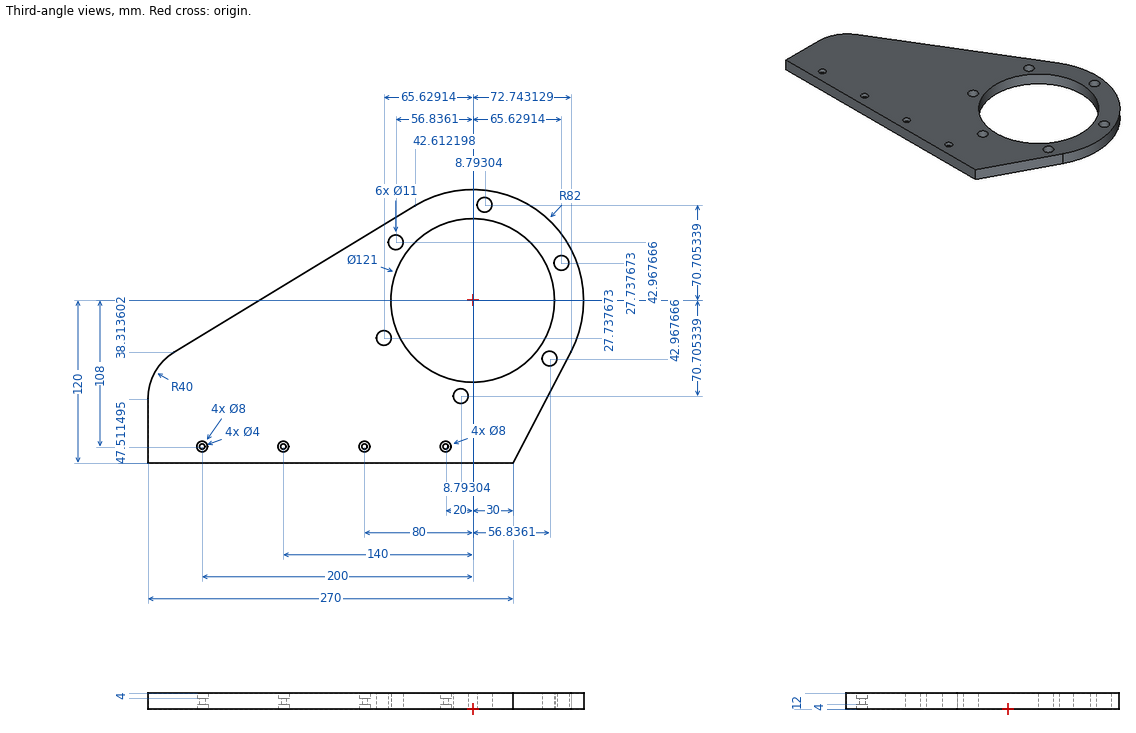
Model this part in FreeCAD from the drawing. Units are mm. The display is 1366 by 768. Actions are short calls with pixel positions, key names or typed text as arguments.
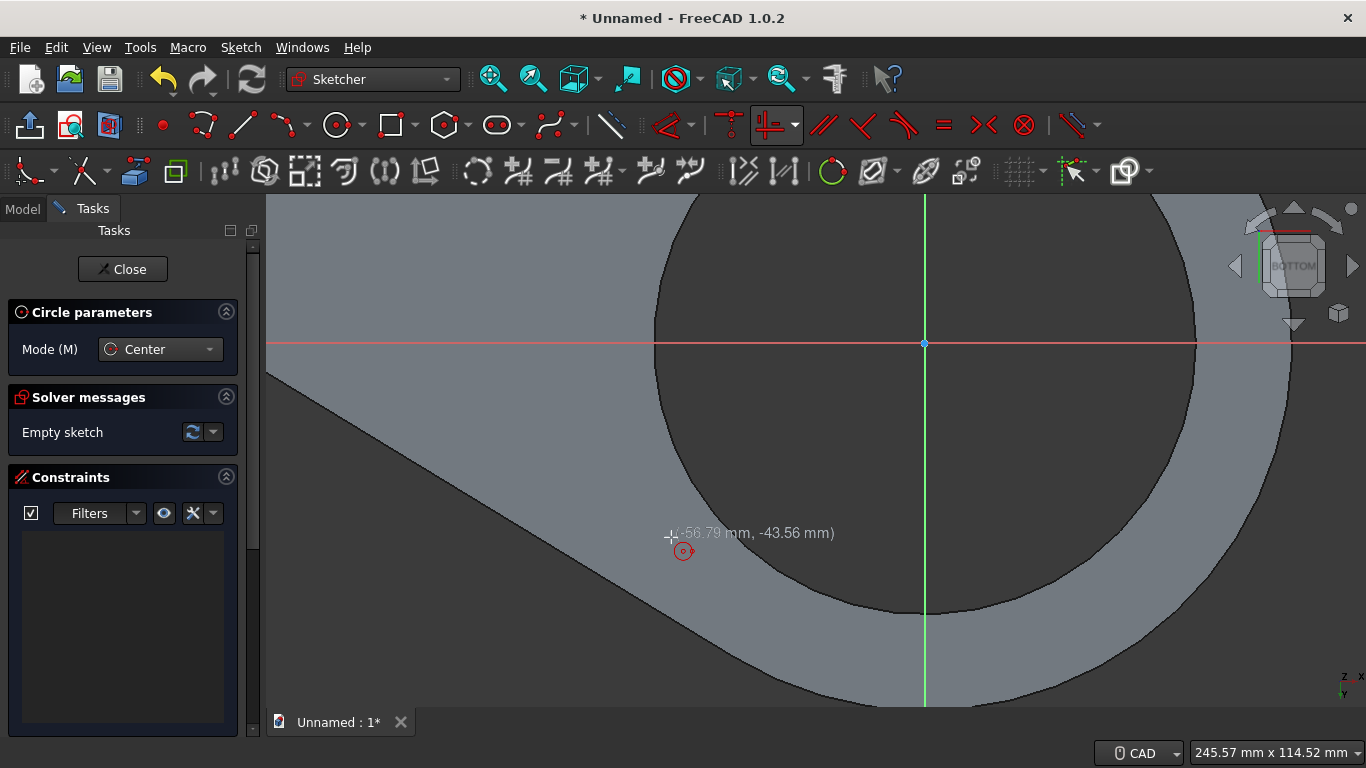
click(670, 536)
click(688, 518)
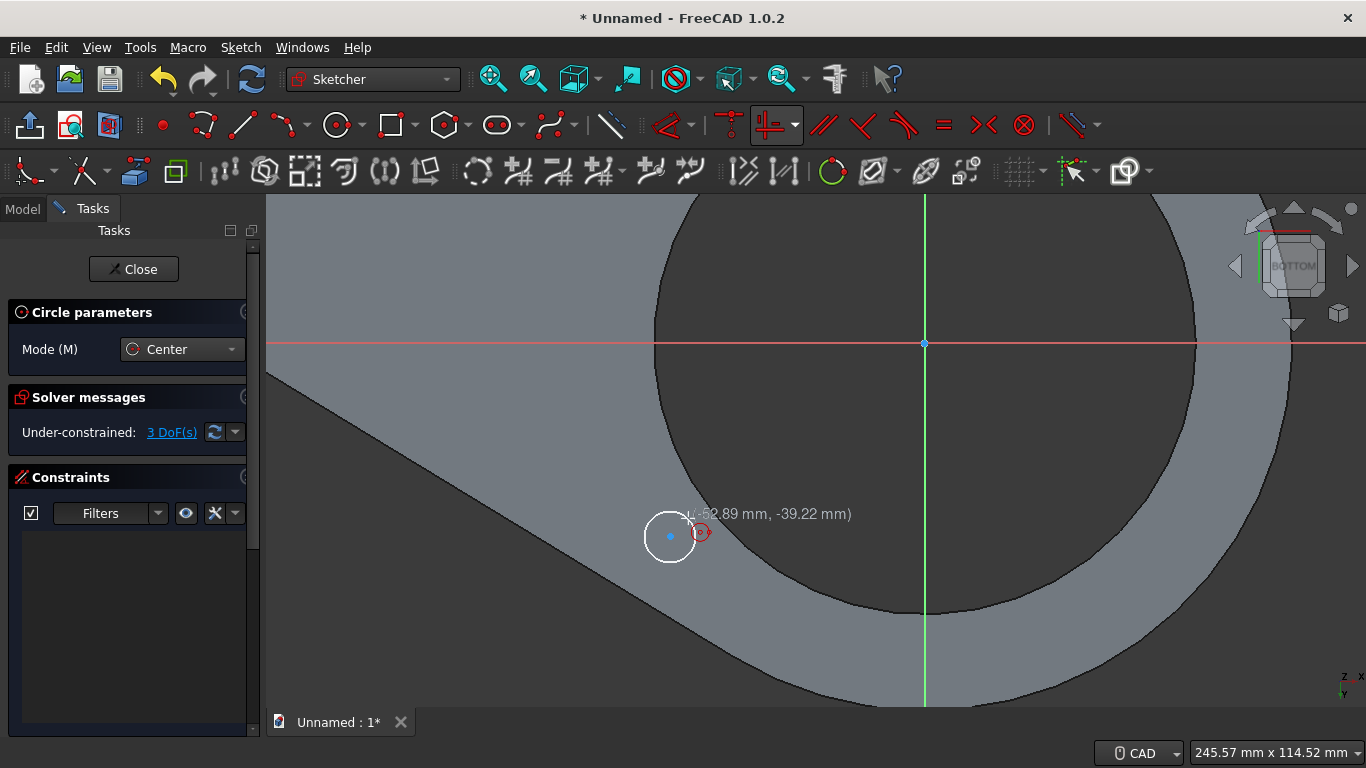
click(964, 660)
click(982, 643)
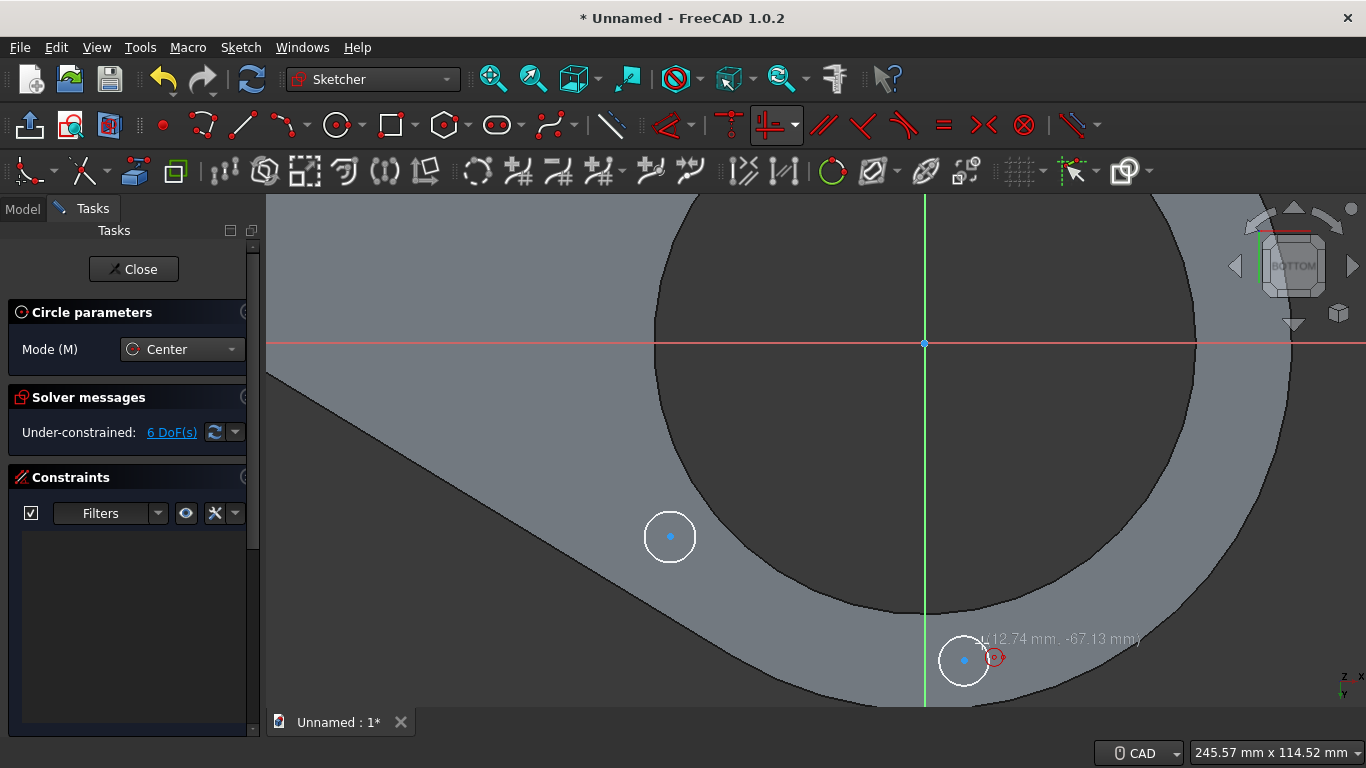
scroll(603, 538, down, 4)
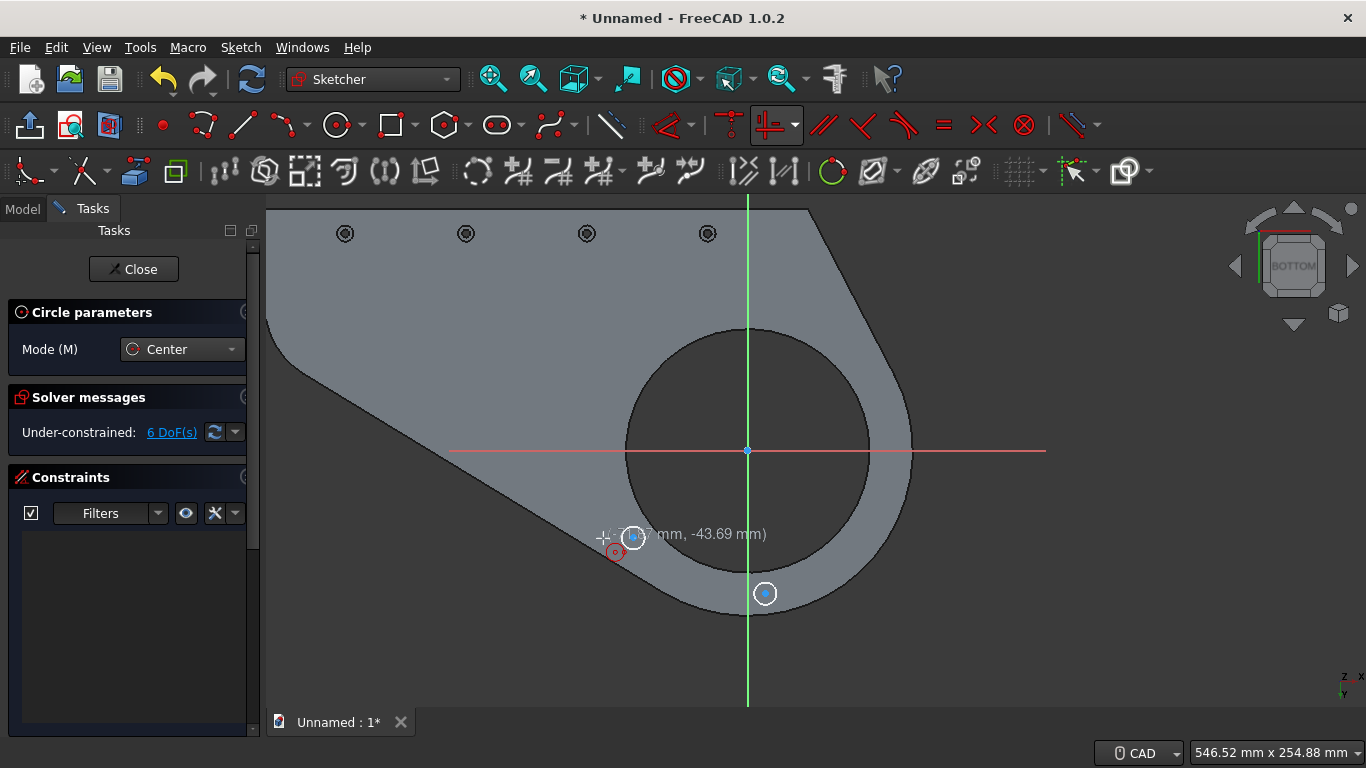
scroll(616, 395, up, 4)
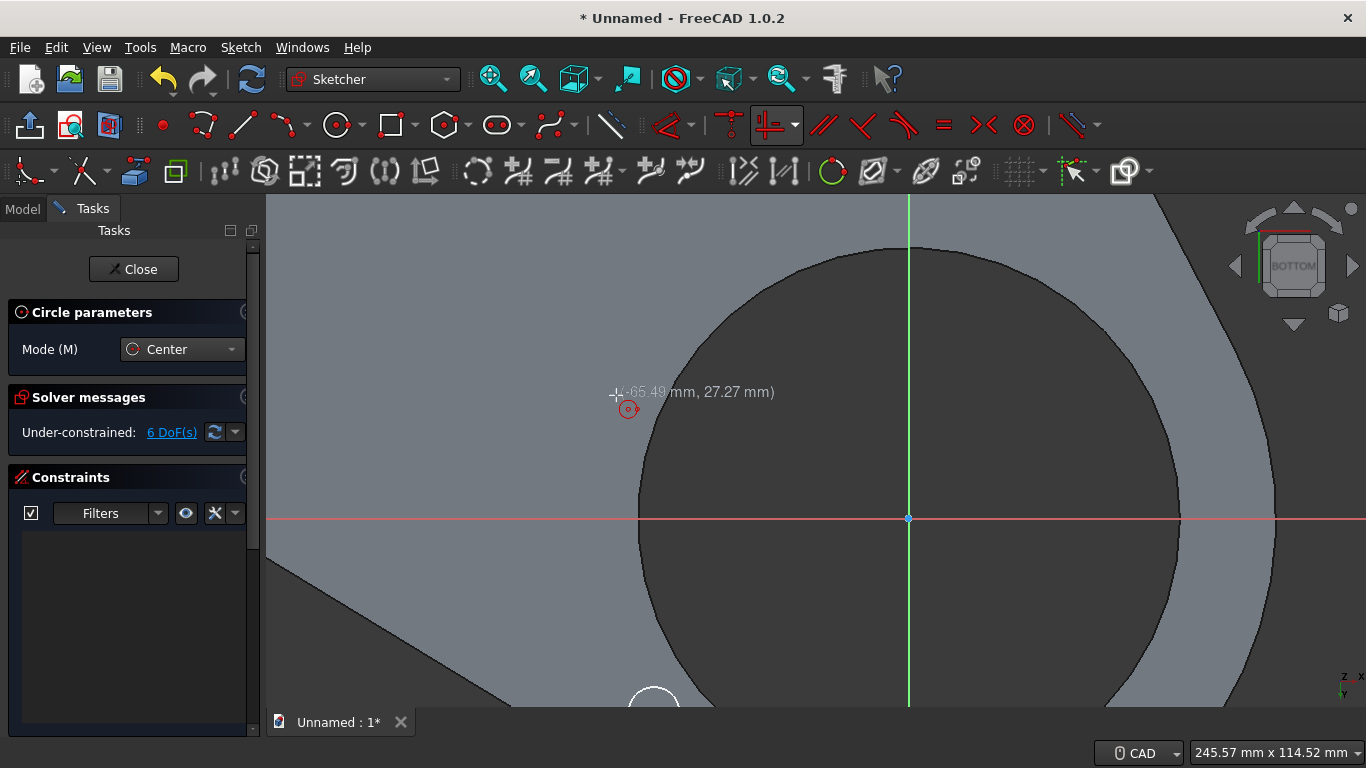
click(615, 395)
click(632, 377)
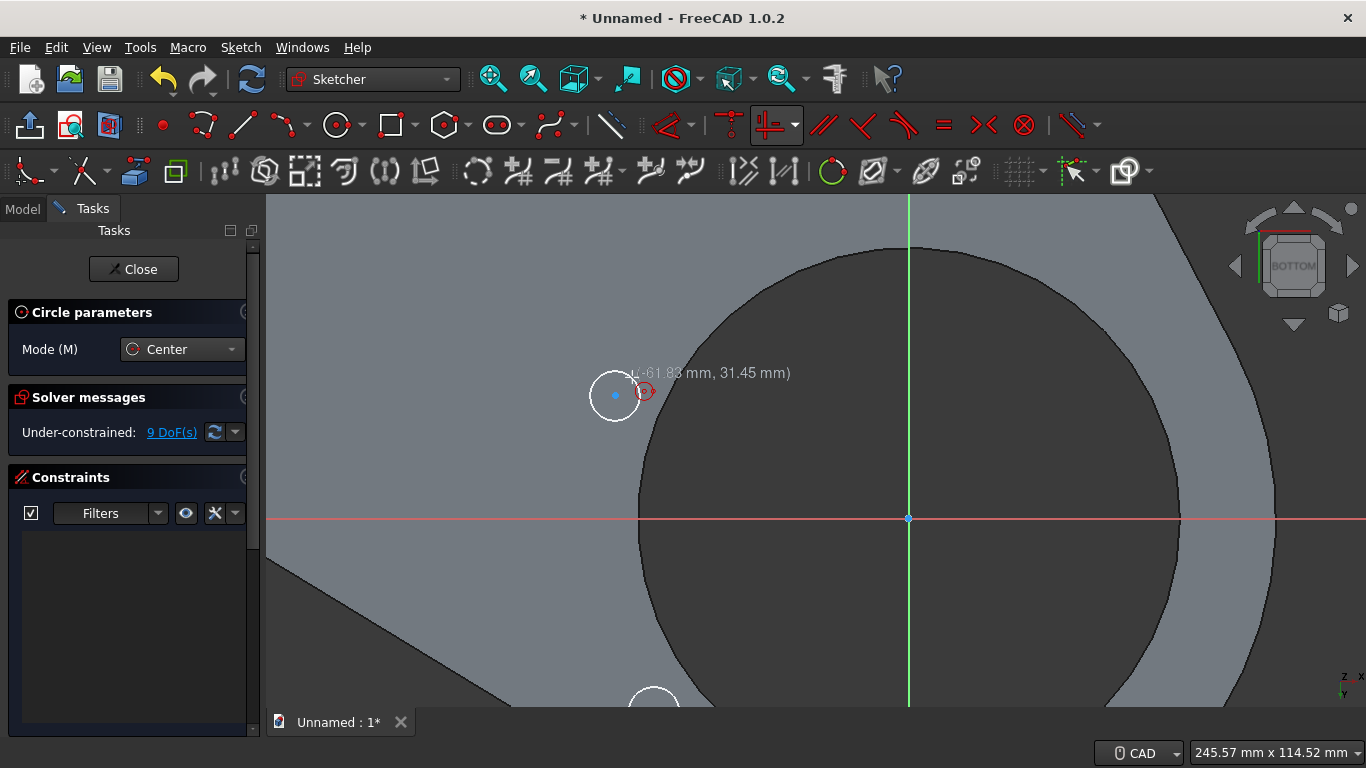
scroll(616, 395, down, 4)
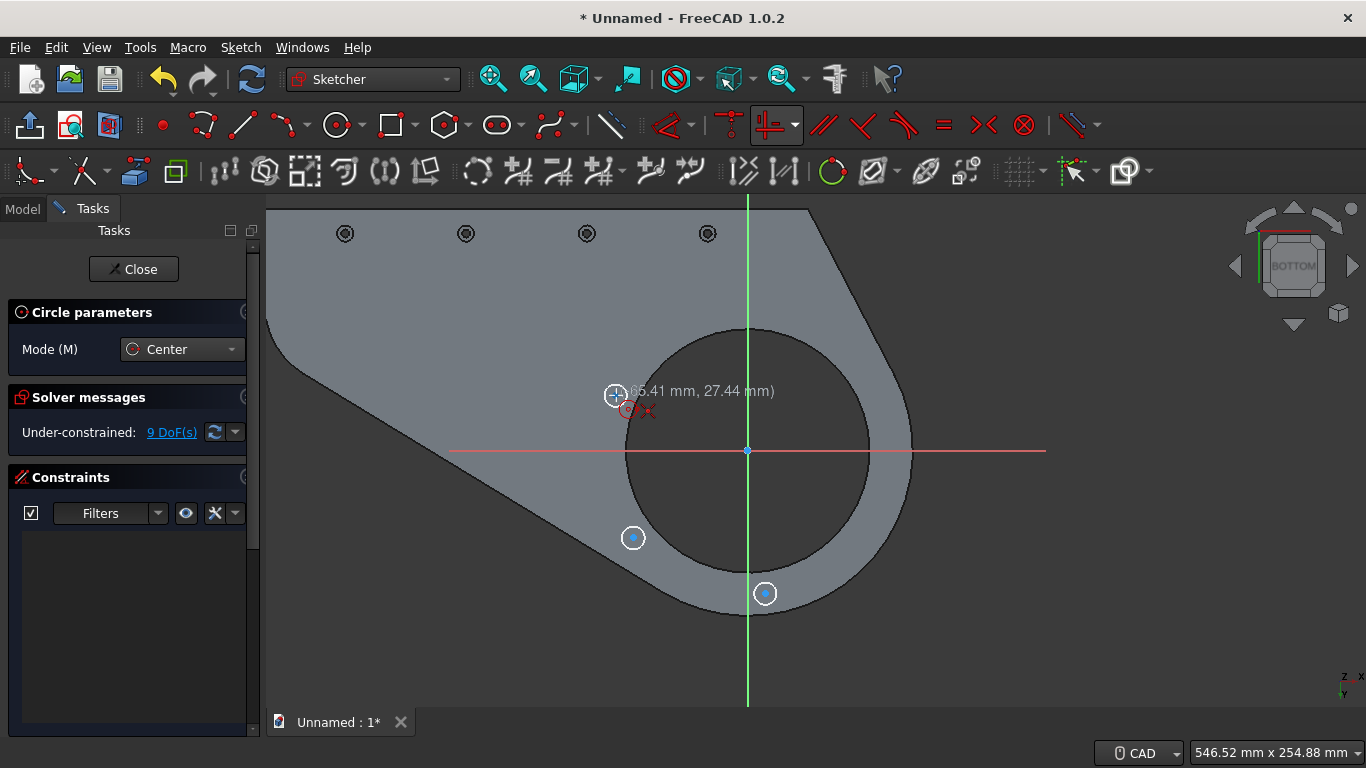
scroll(730, 309, up, 4)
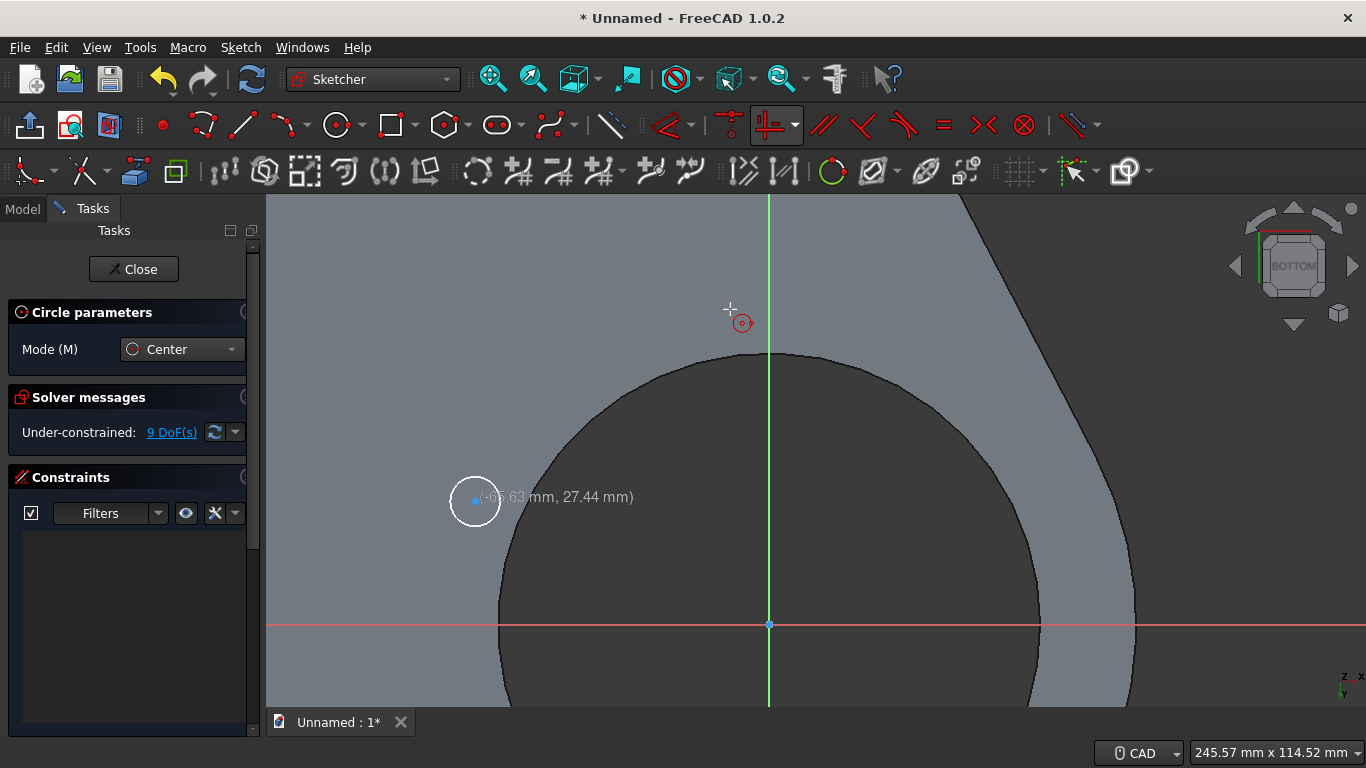
click(730, 308)
click(747, 290)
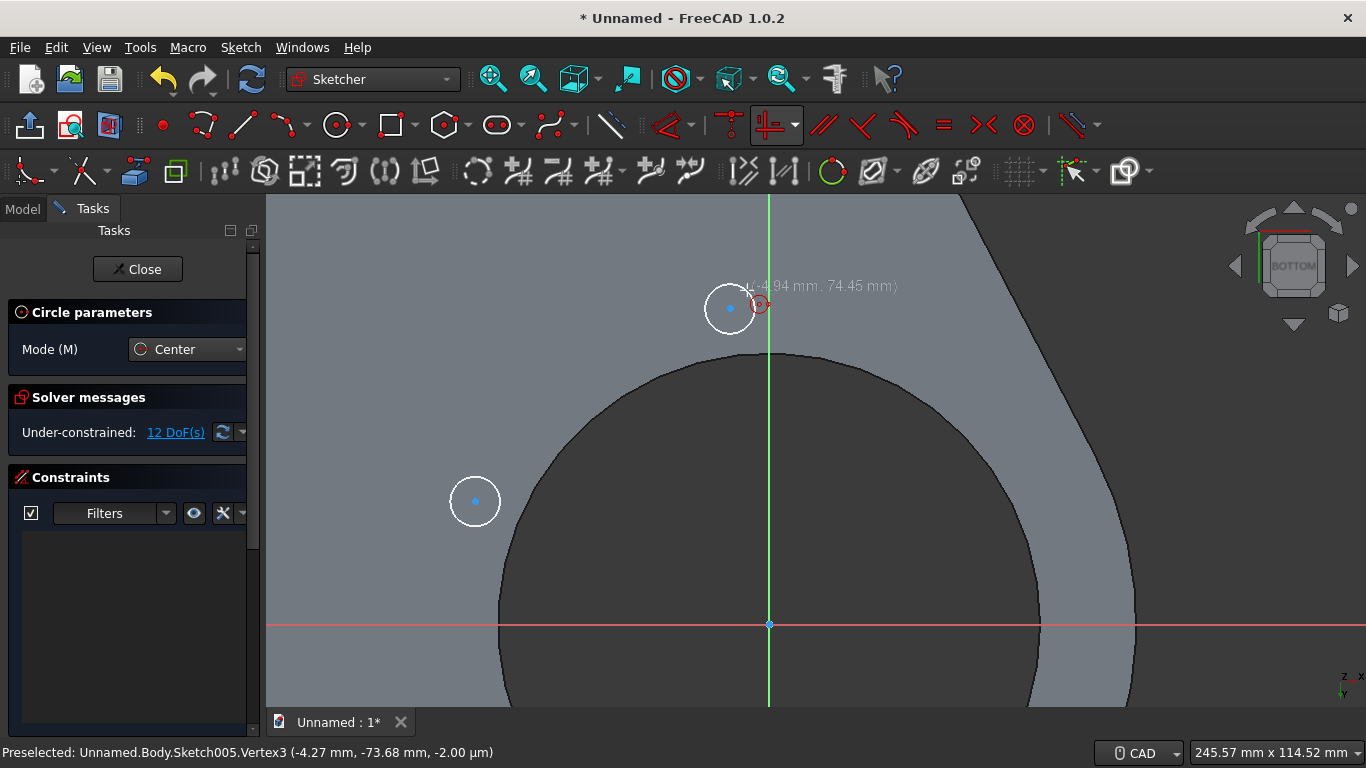
click(1024, 432)
click(1041, 415)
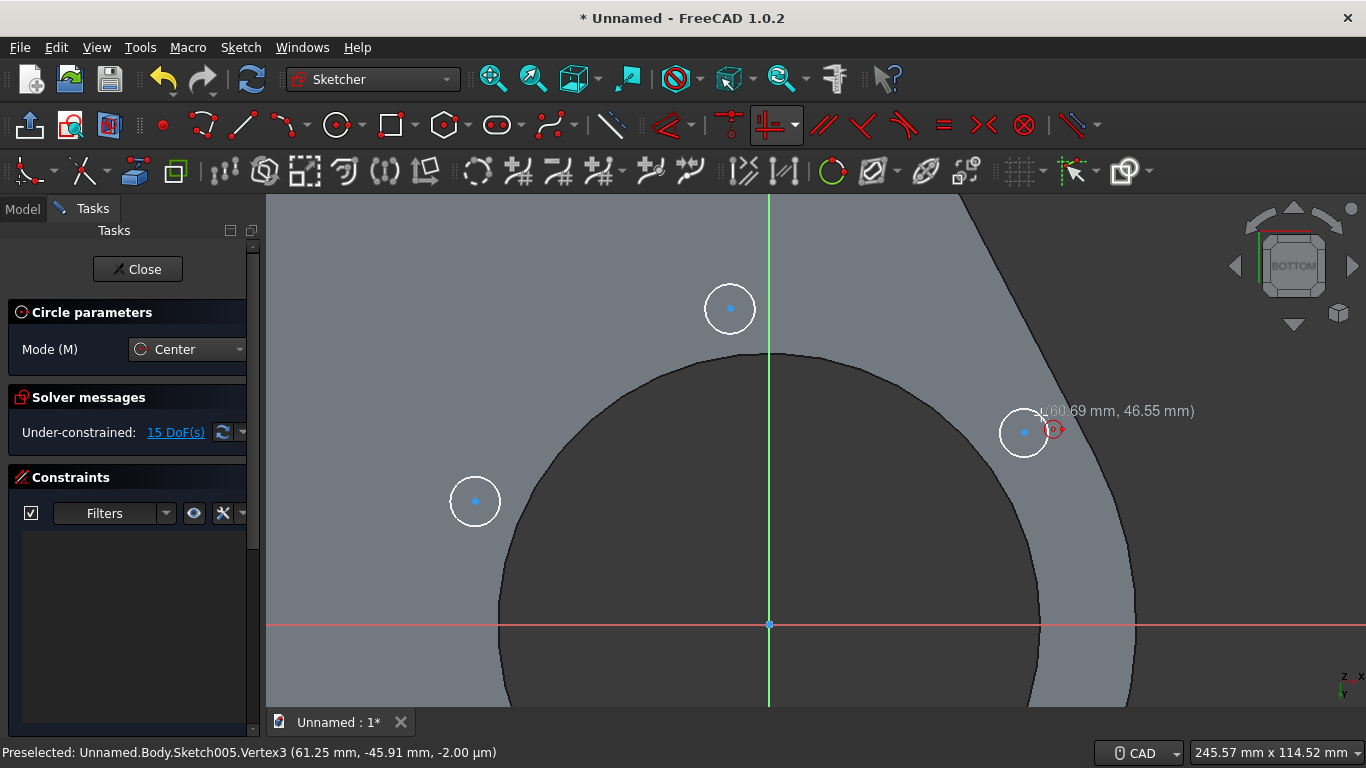
scroll(730, 309, down, 4)